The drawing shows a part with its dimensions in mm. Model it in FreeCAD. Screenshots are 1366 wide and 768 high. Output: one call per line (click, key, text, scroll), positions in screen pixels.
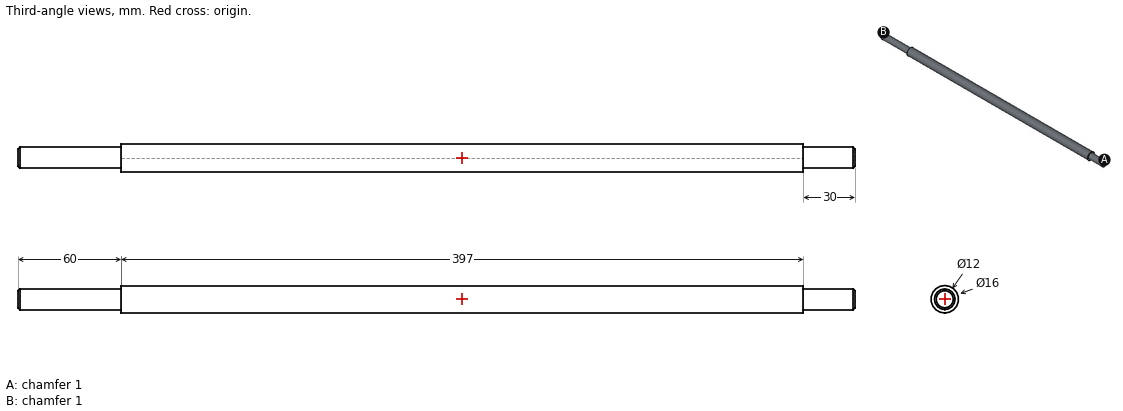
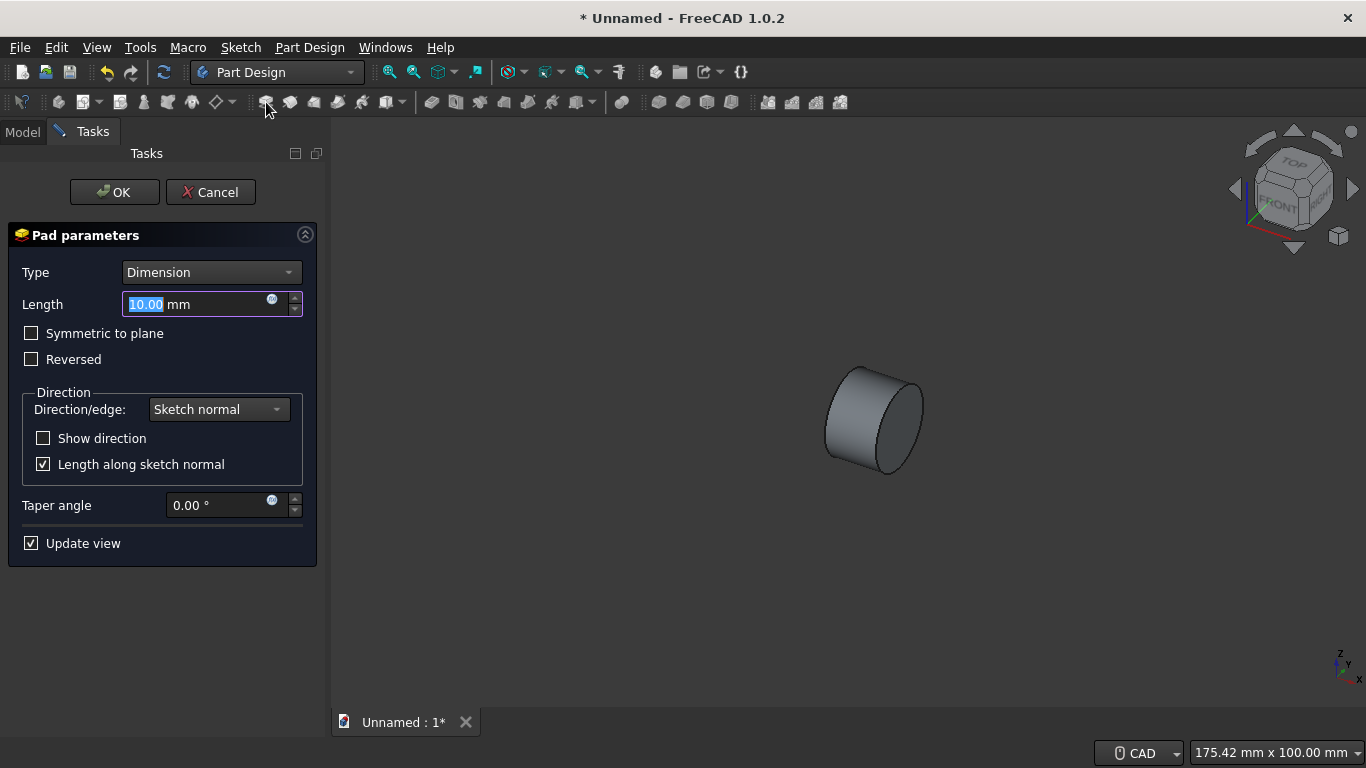
text(397)
key(Tab)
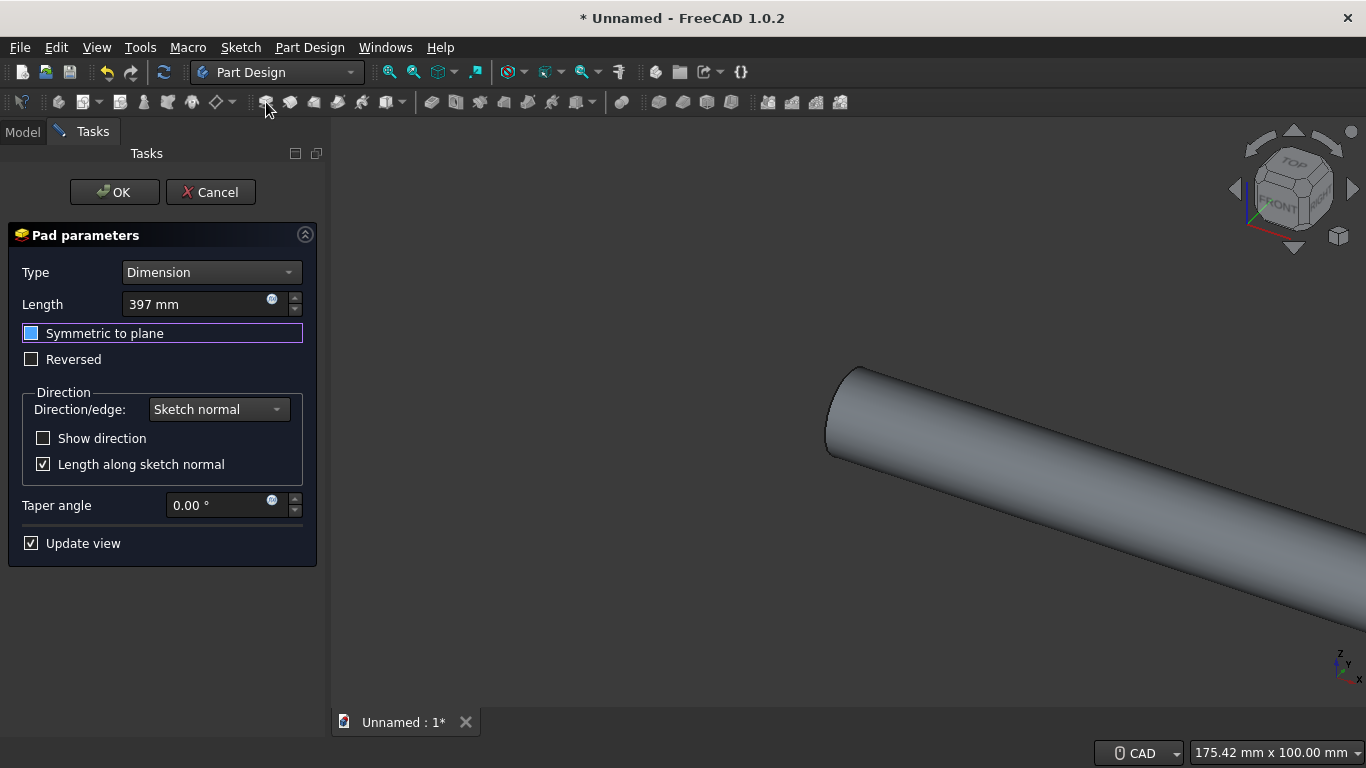
click(30, 333)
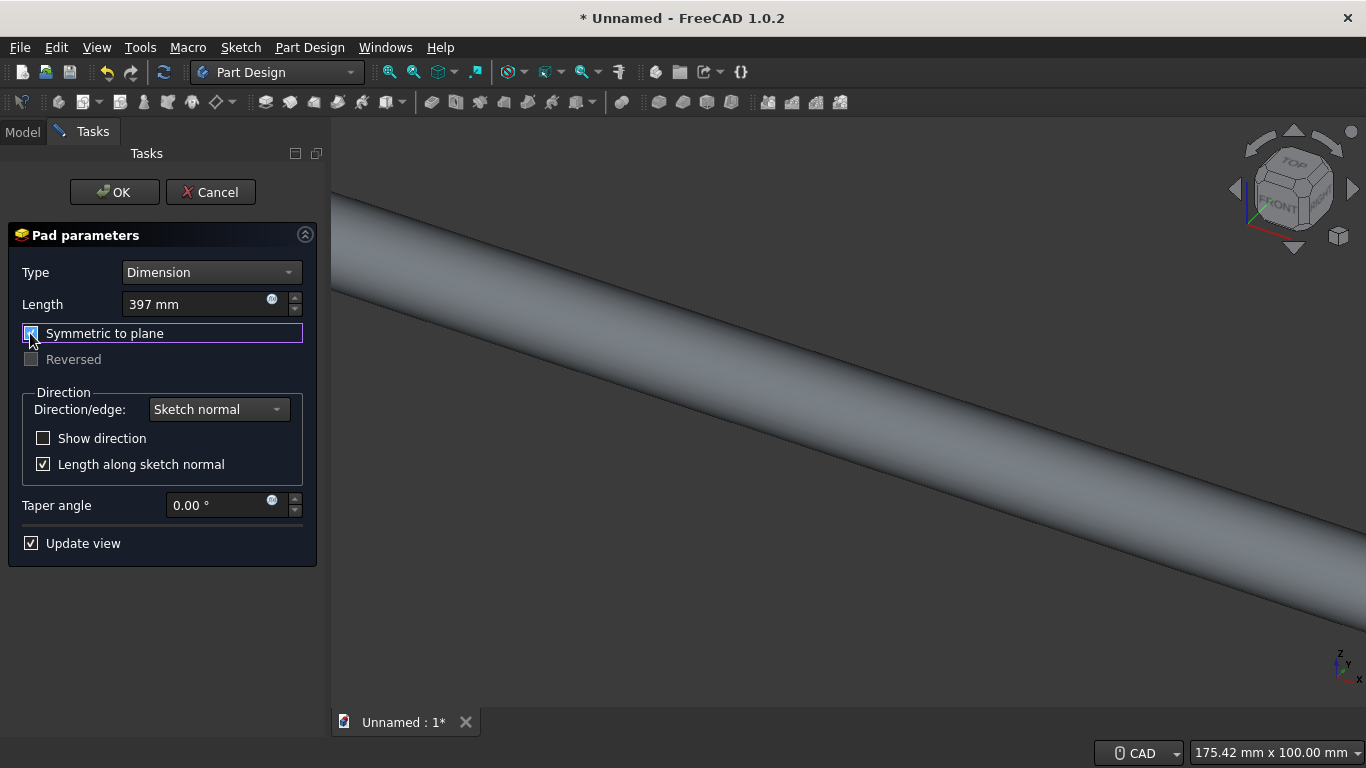
click(115, 192)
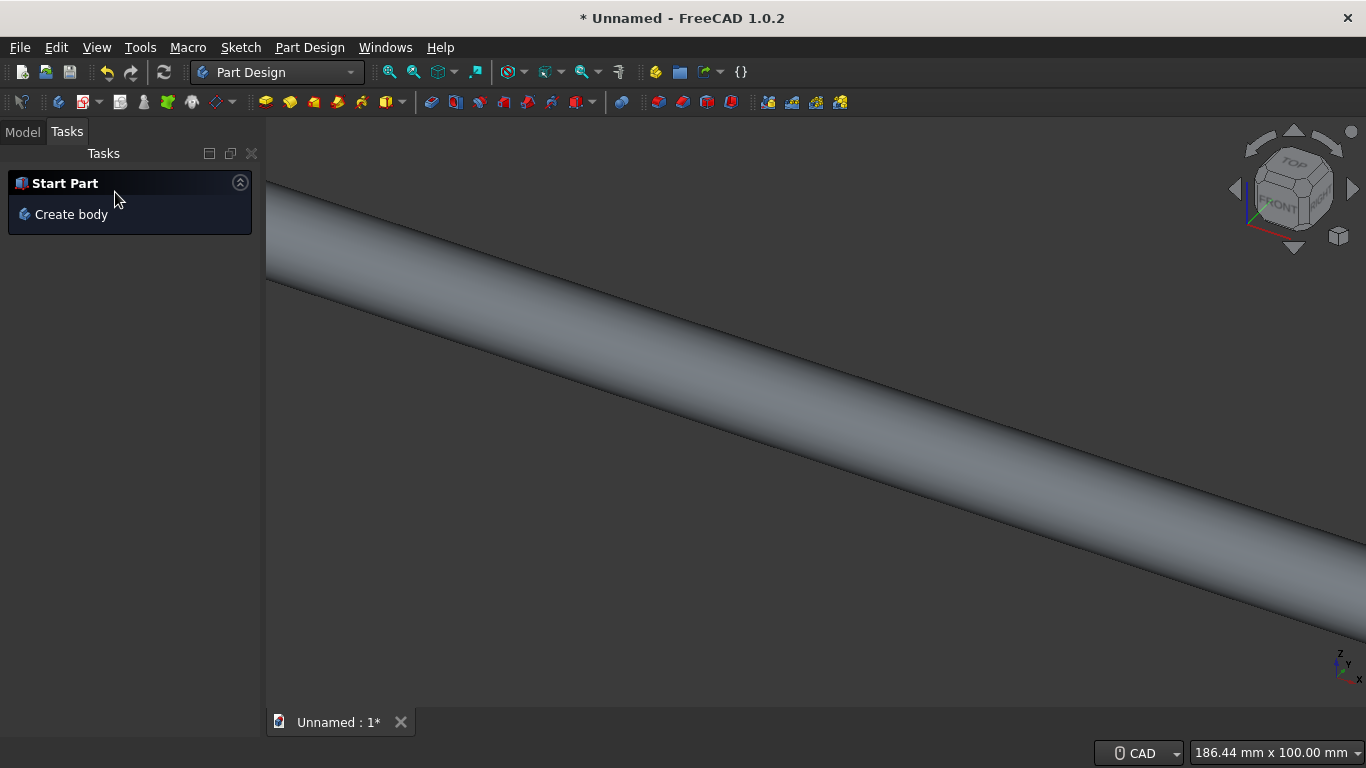
click(390, 72)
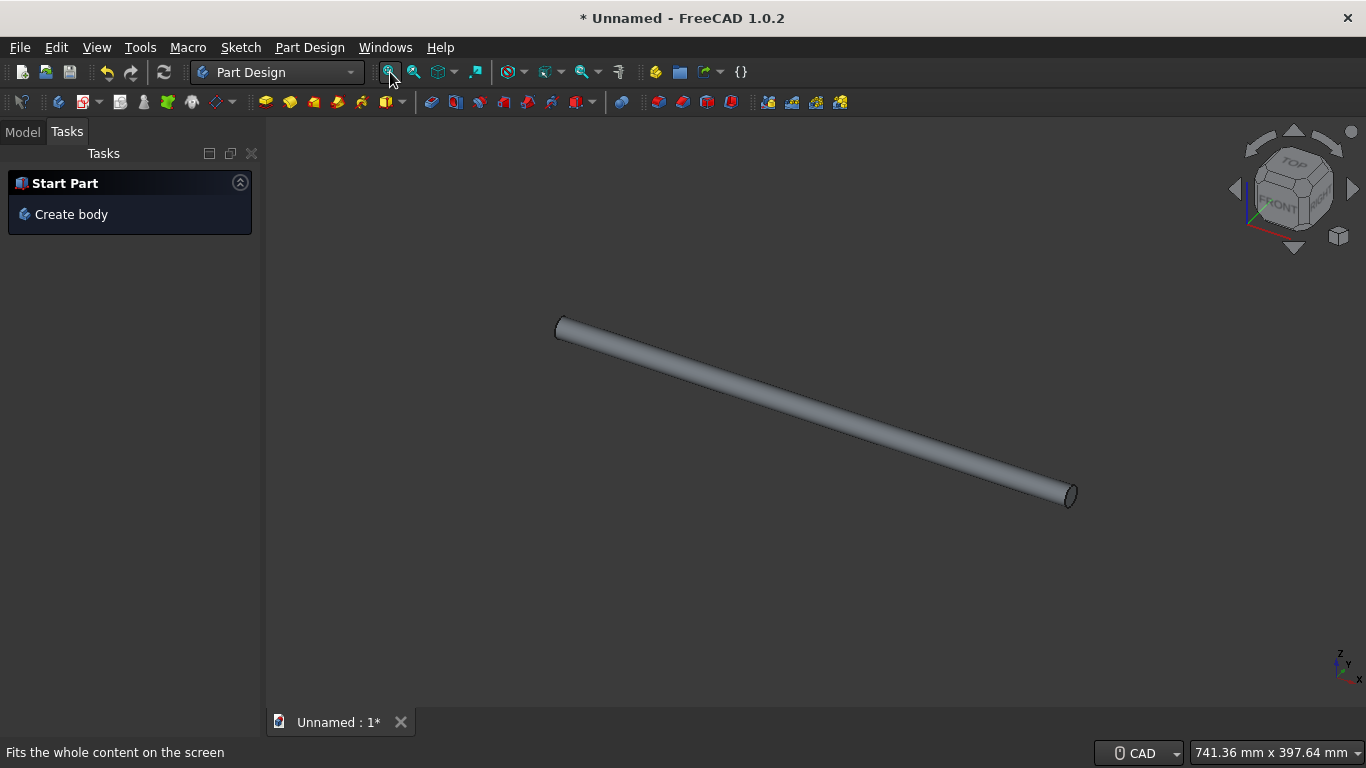
key(0)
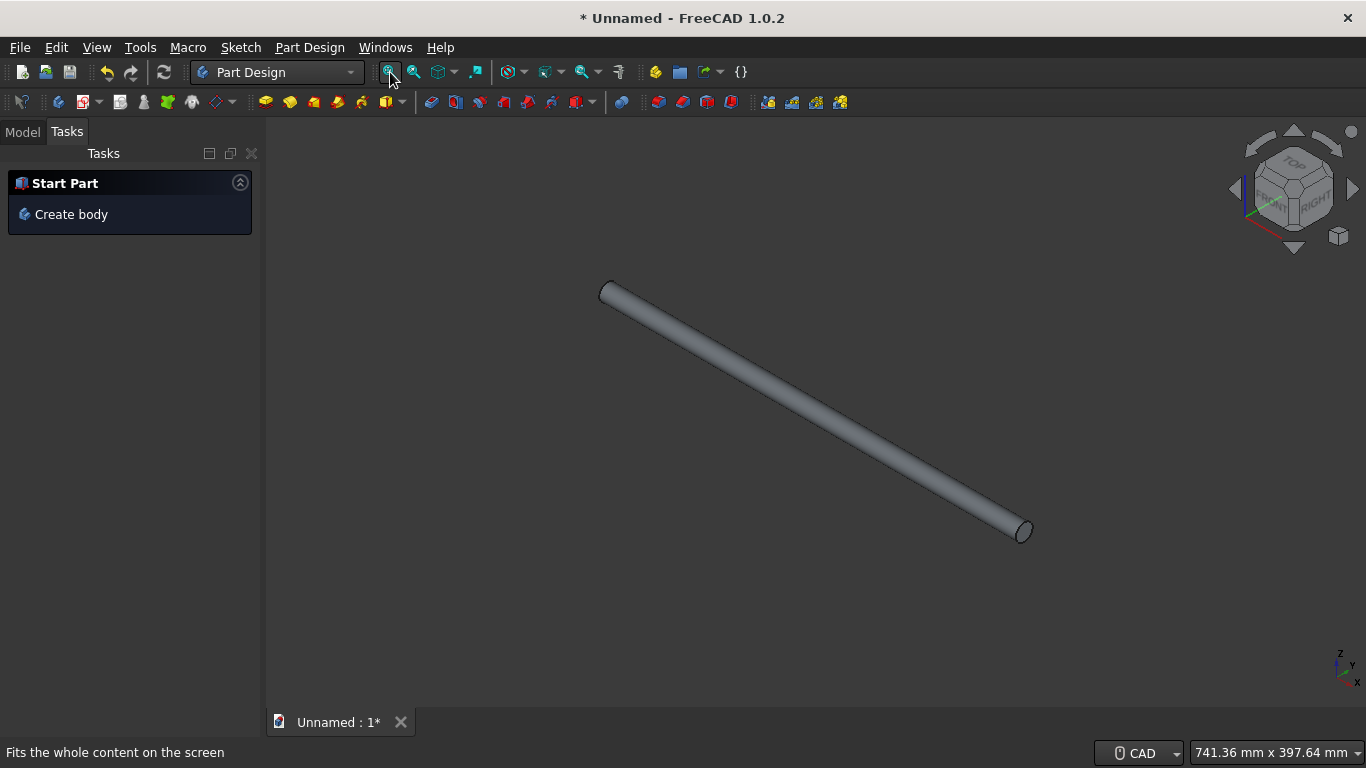
key(3)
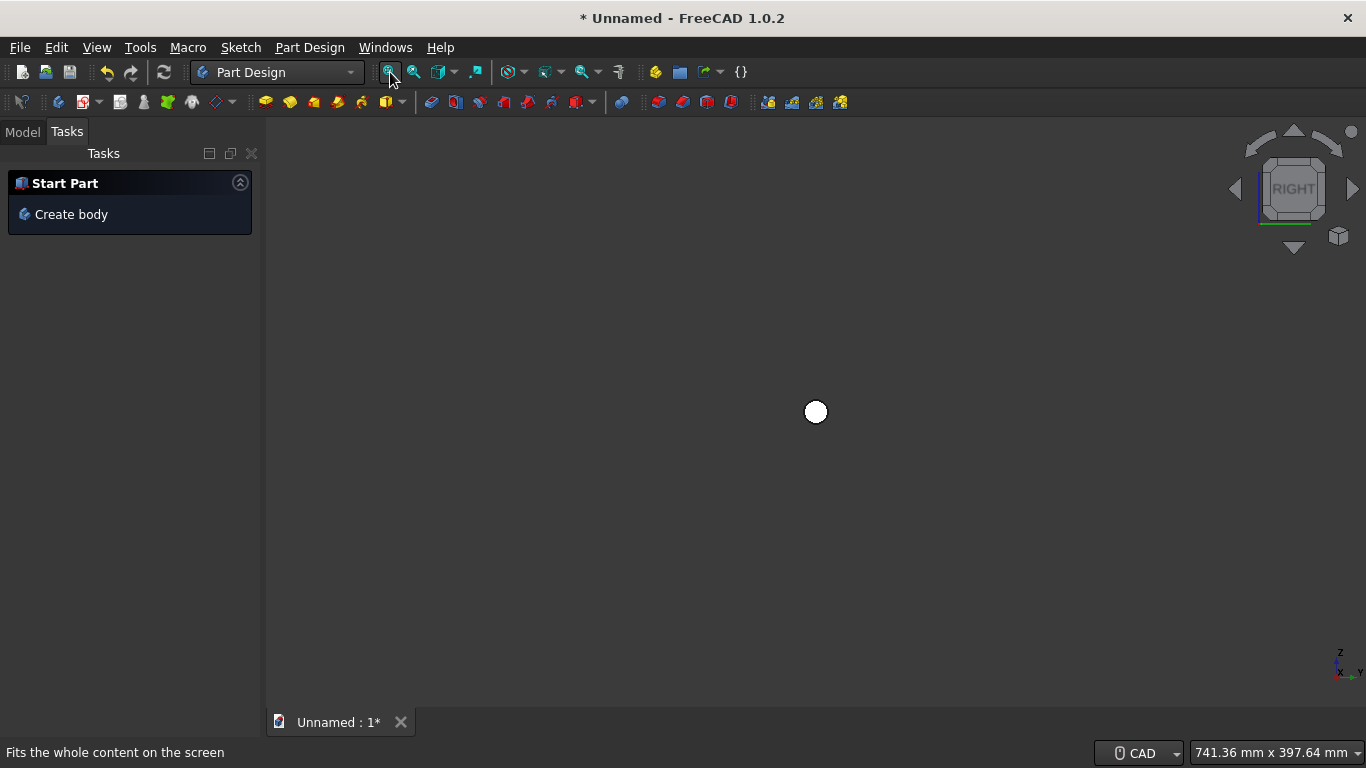
click(390, 72)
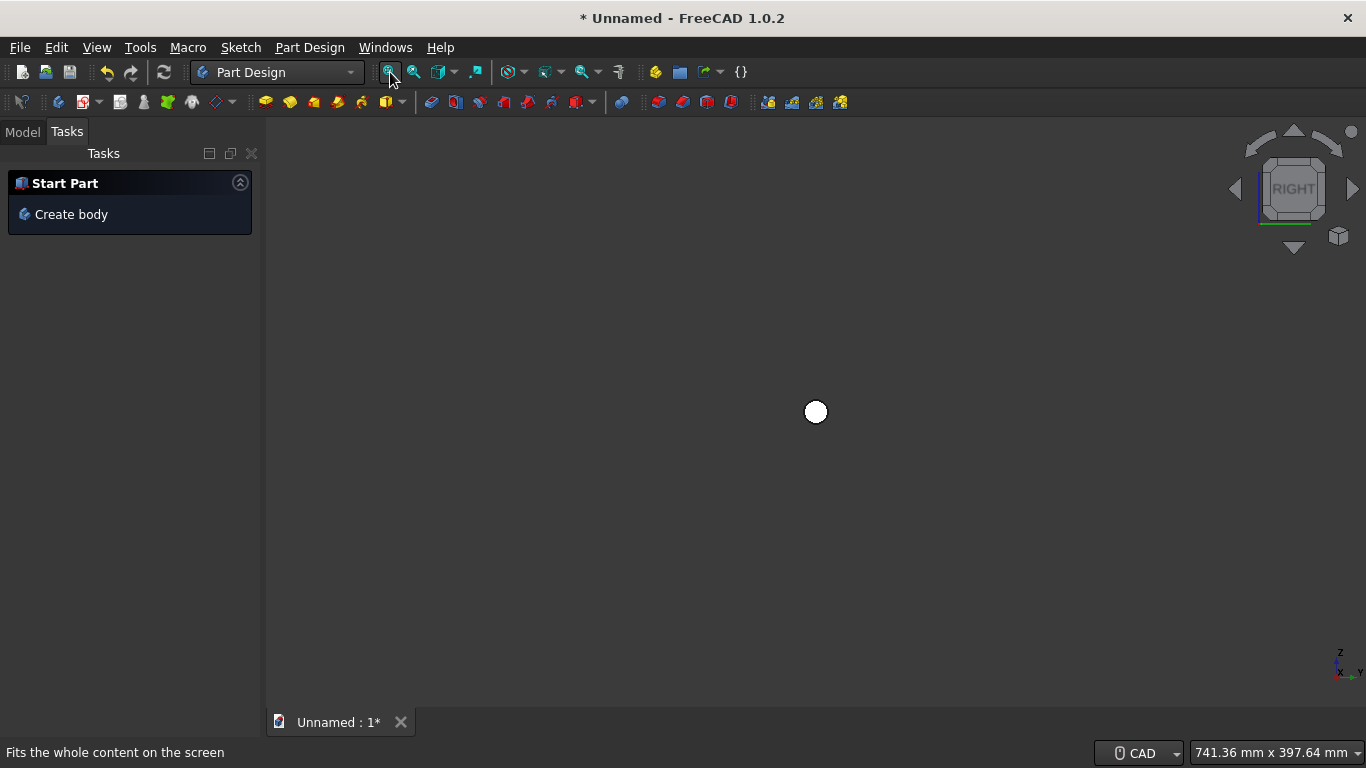
click(816, 411)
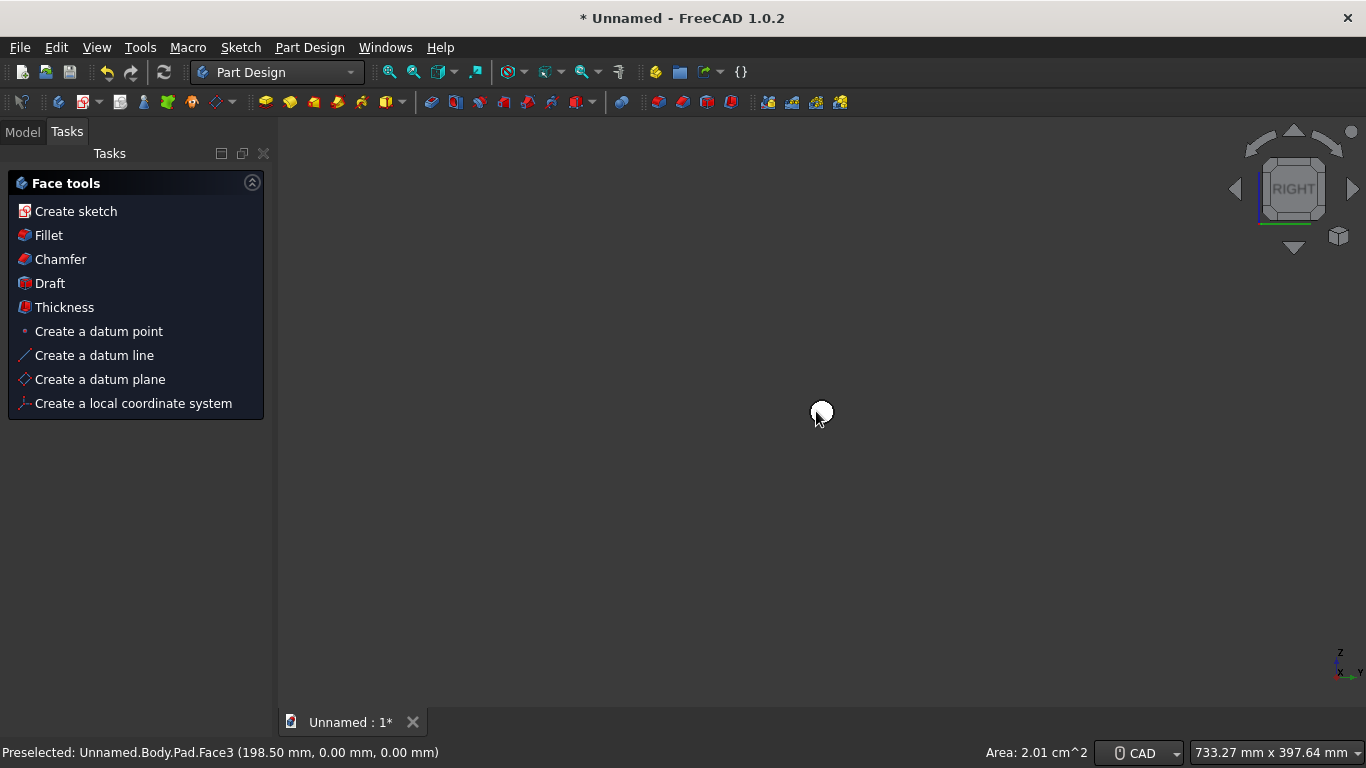
click(84, 102)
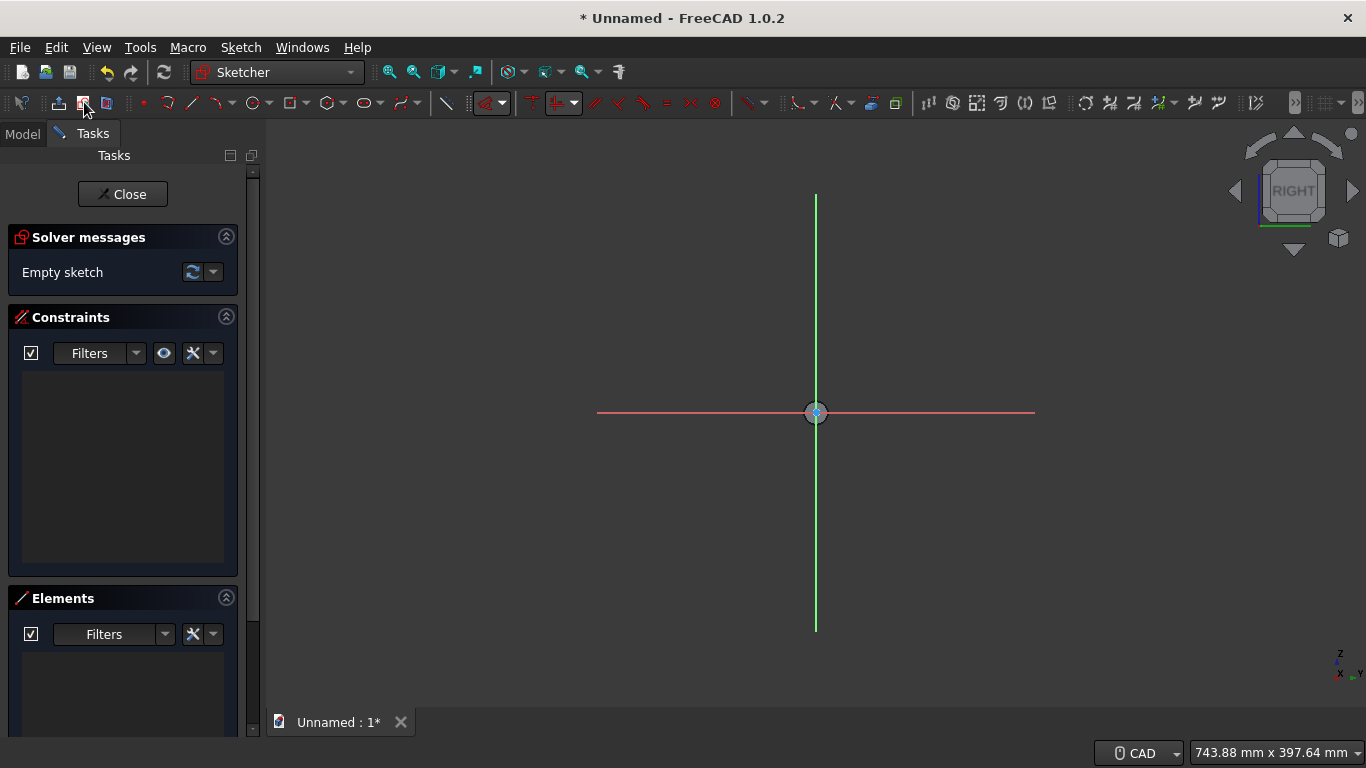
scroll(820, 413, up, 15)